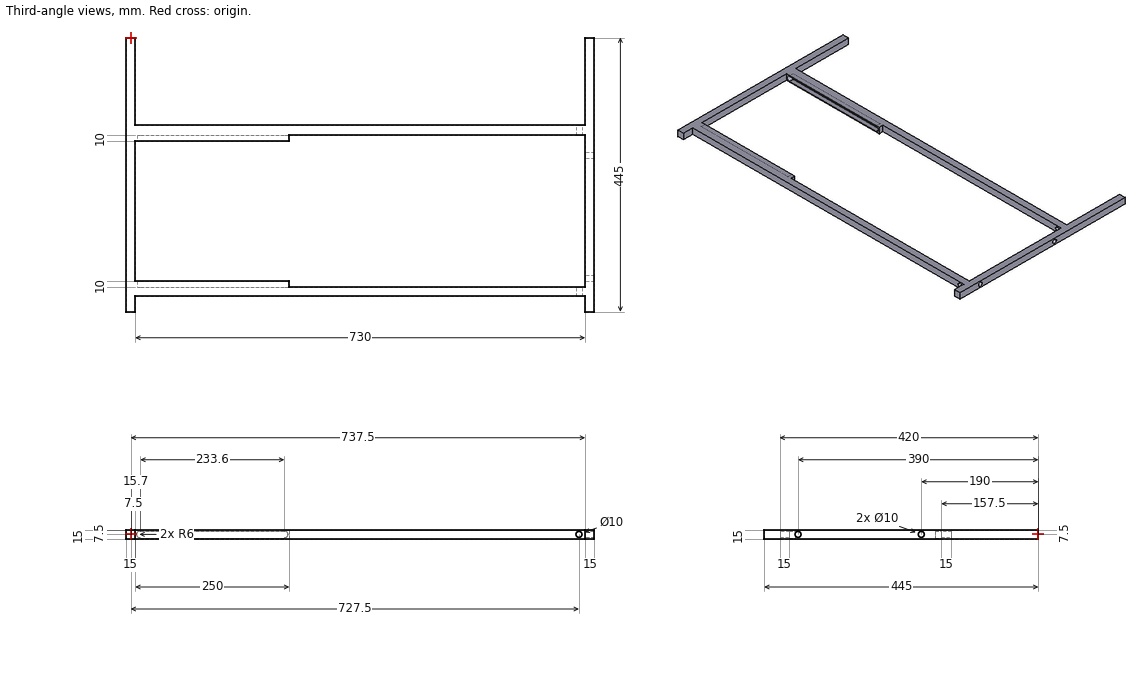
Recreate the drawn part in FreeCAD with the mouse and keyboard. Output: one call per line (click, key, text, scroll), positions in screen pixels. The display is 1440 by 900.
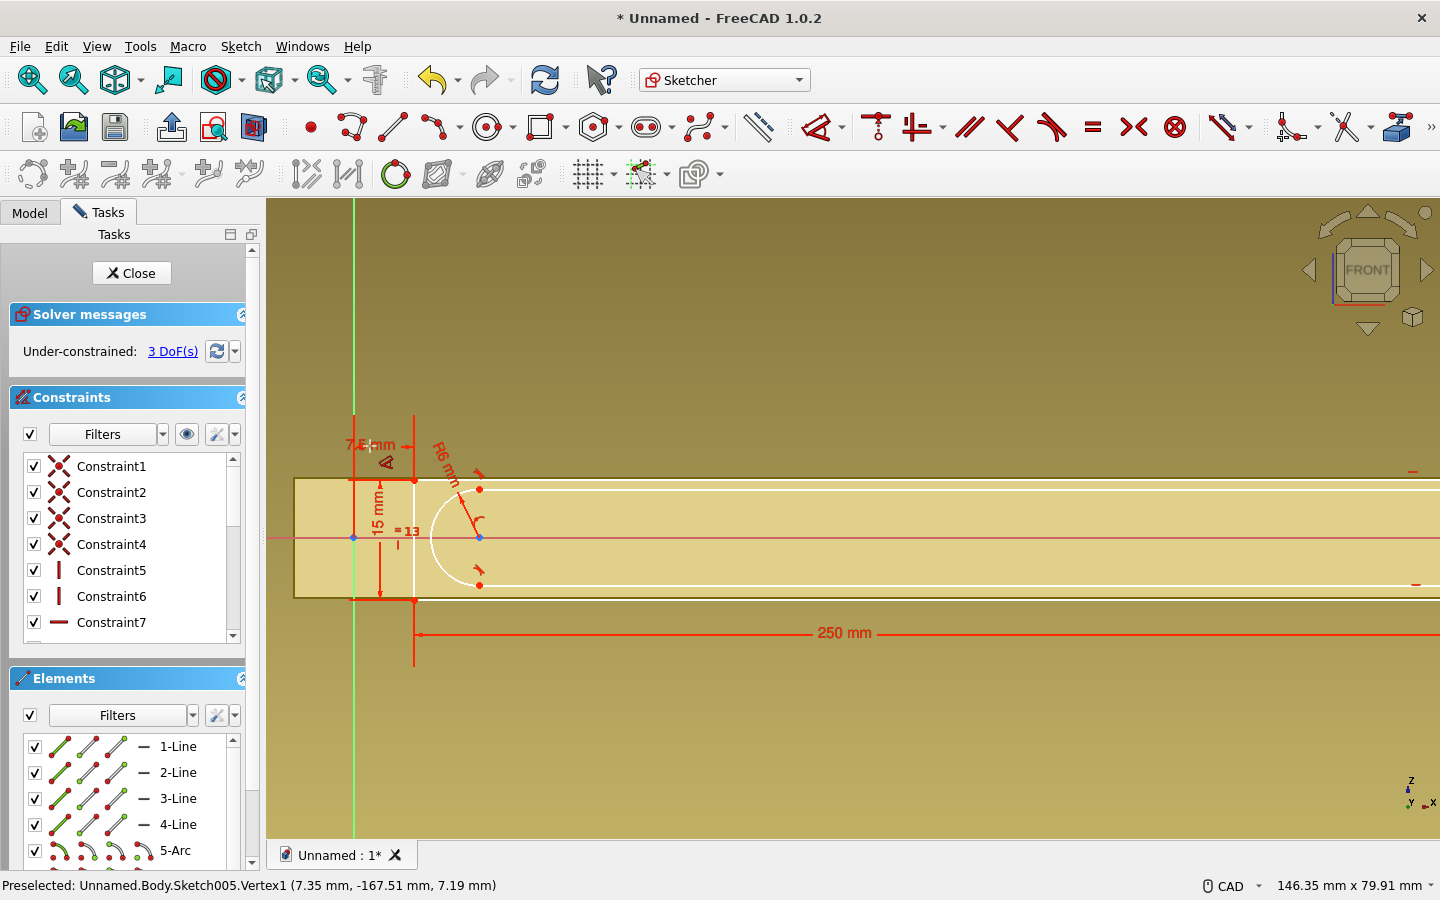
click(414, 480)
click(320, 489)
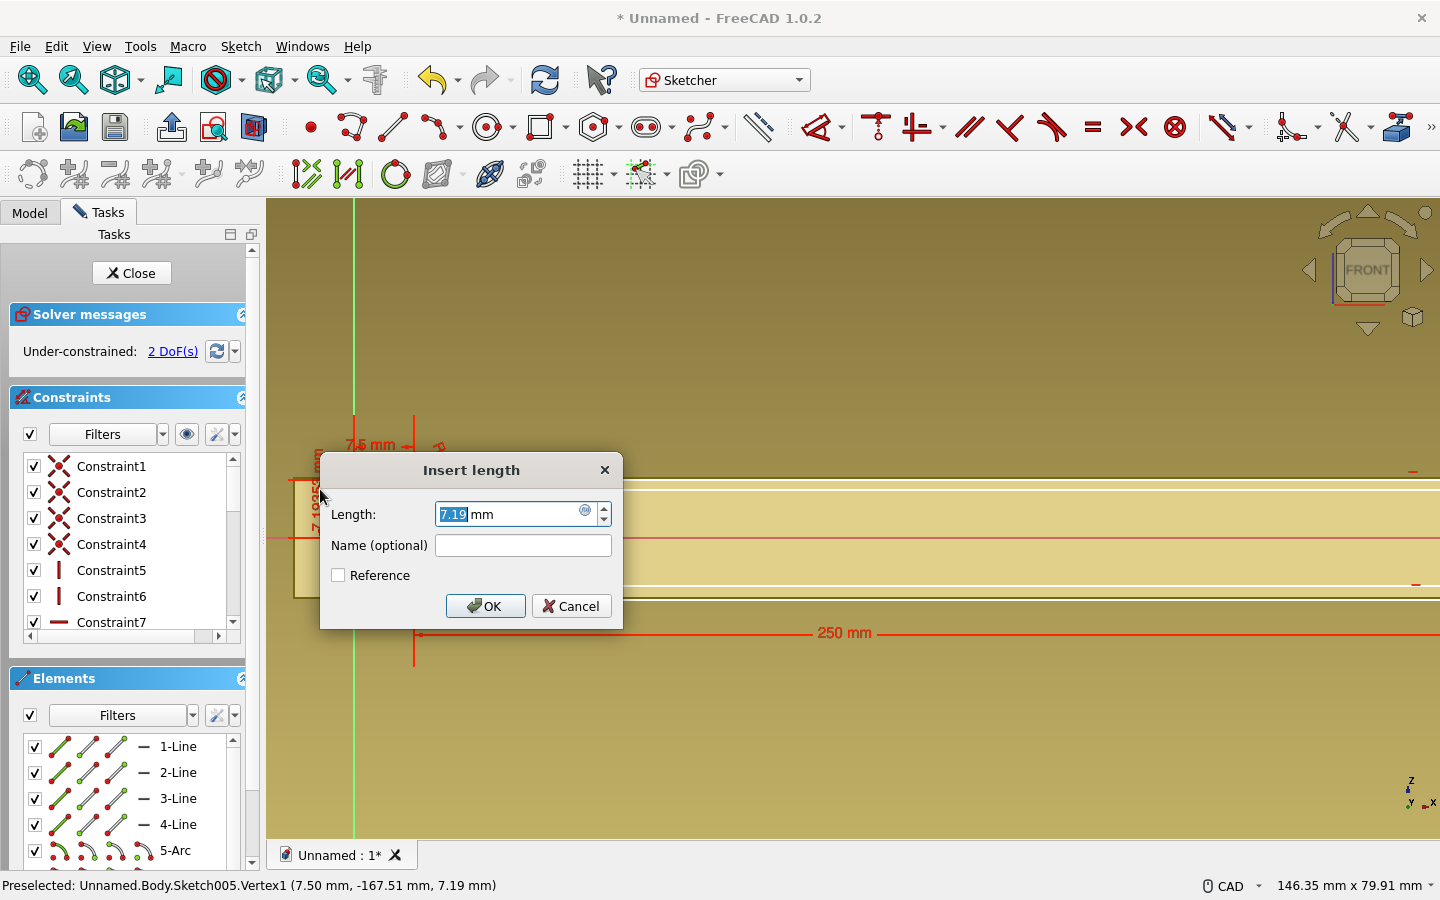
text(7.5)
key(Return)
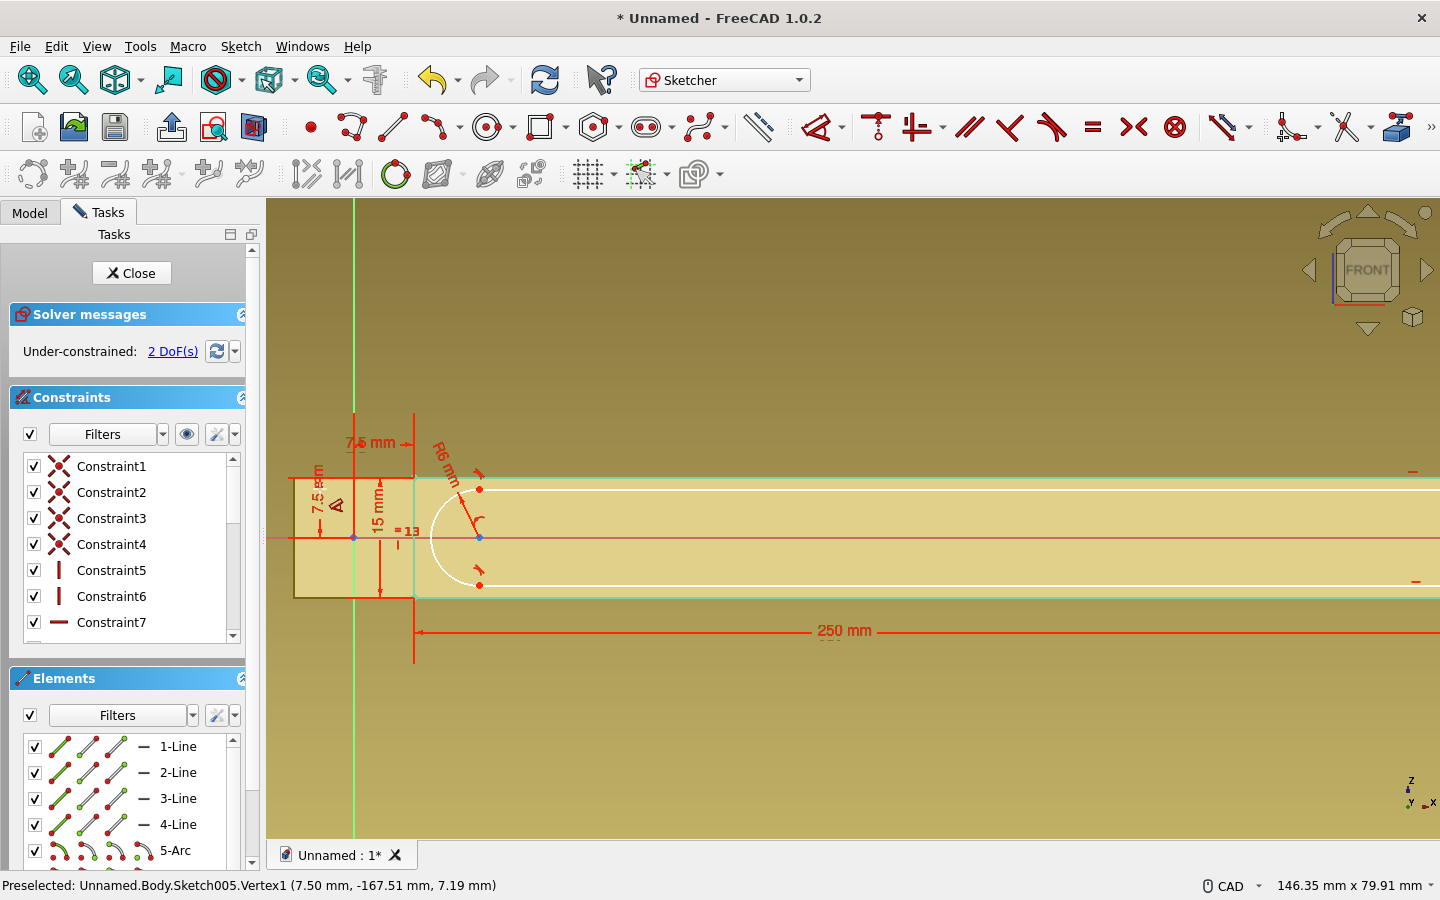
click(1041, 490)
click(877, 456)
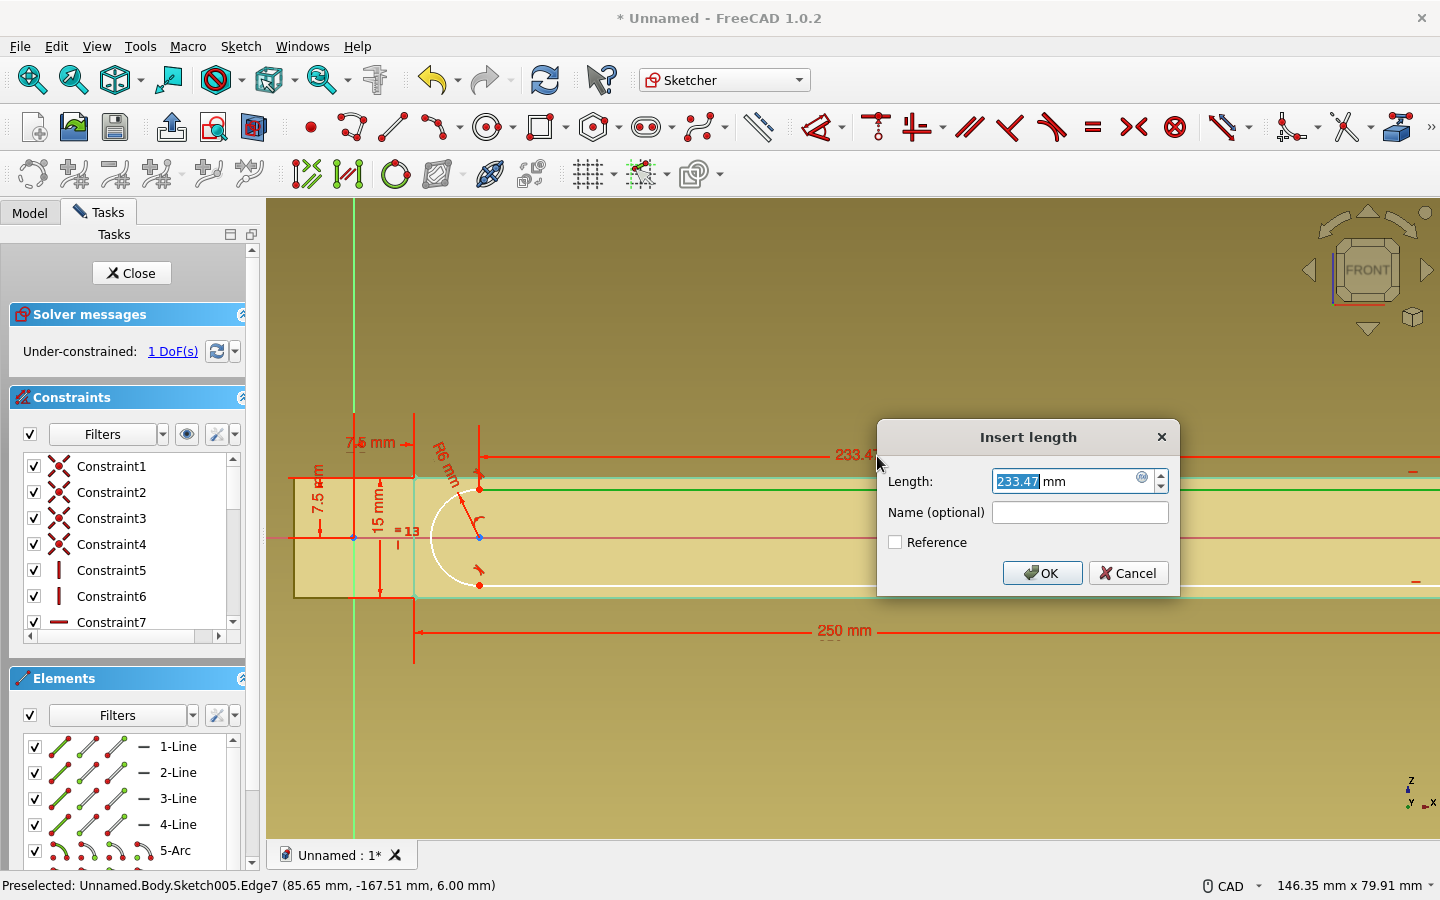
text(233.6)
key(Return)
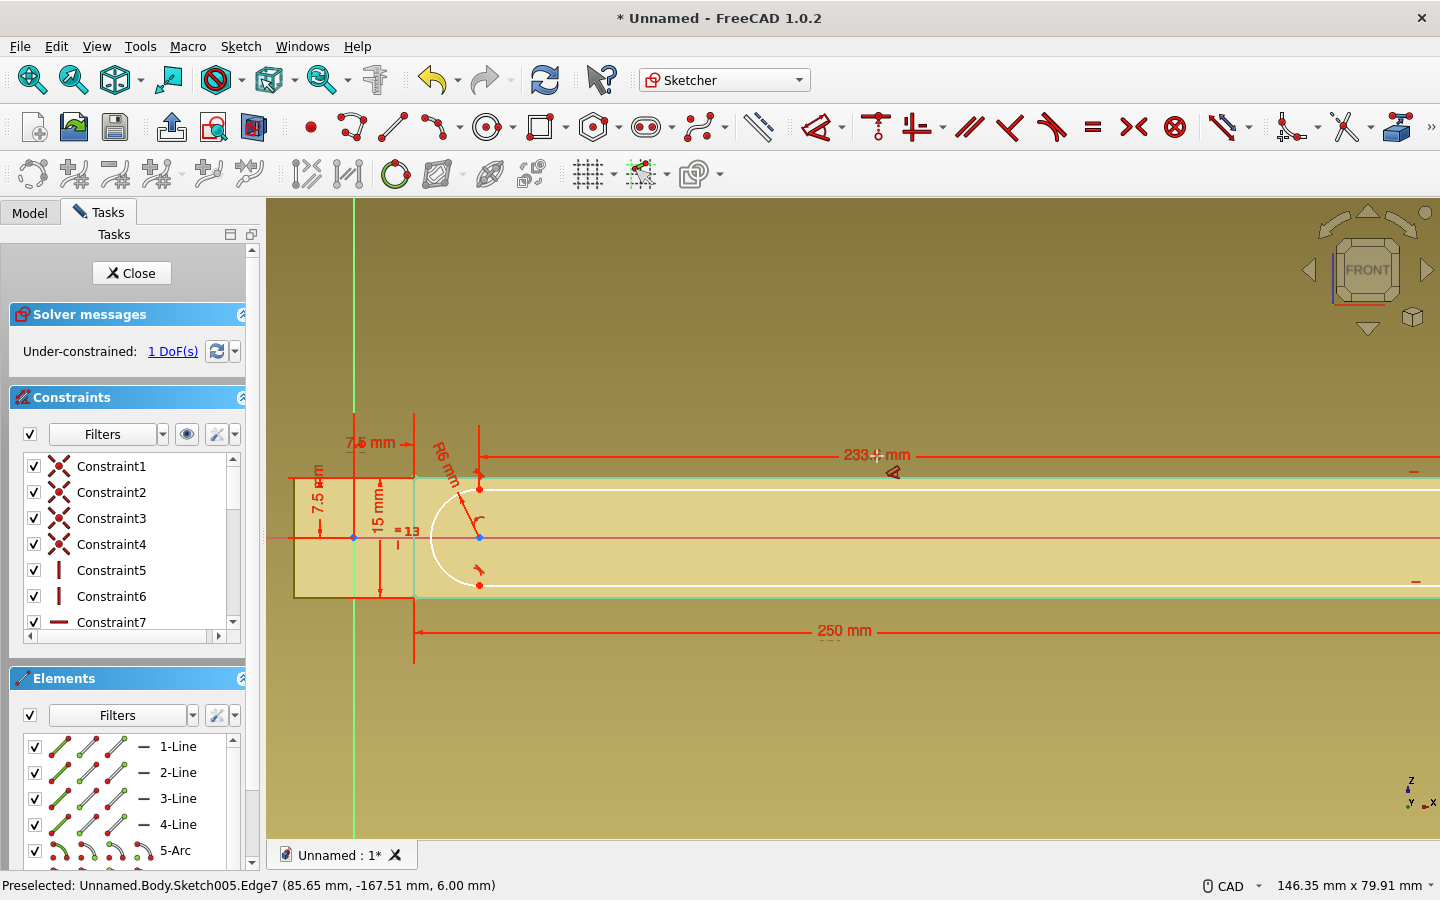
click(479, 490)
click(388, 572)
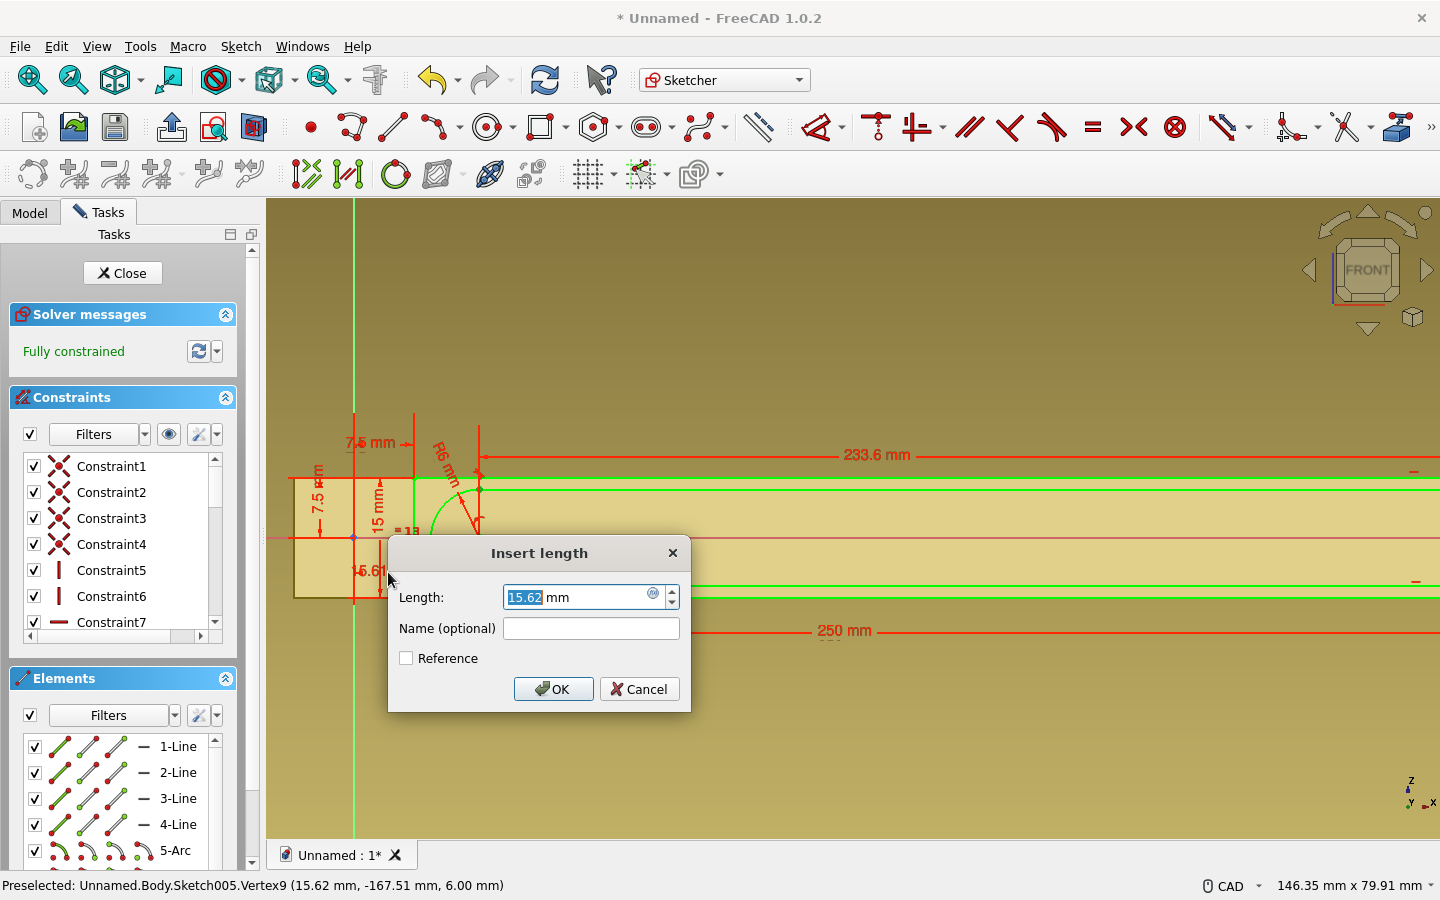
text(15.7)
key(Return)
key(Escape)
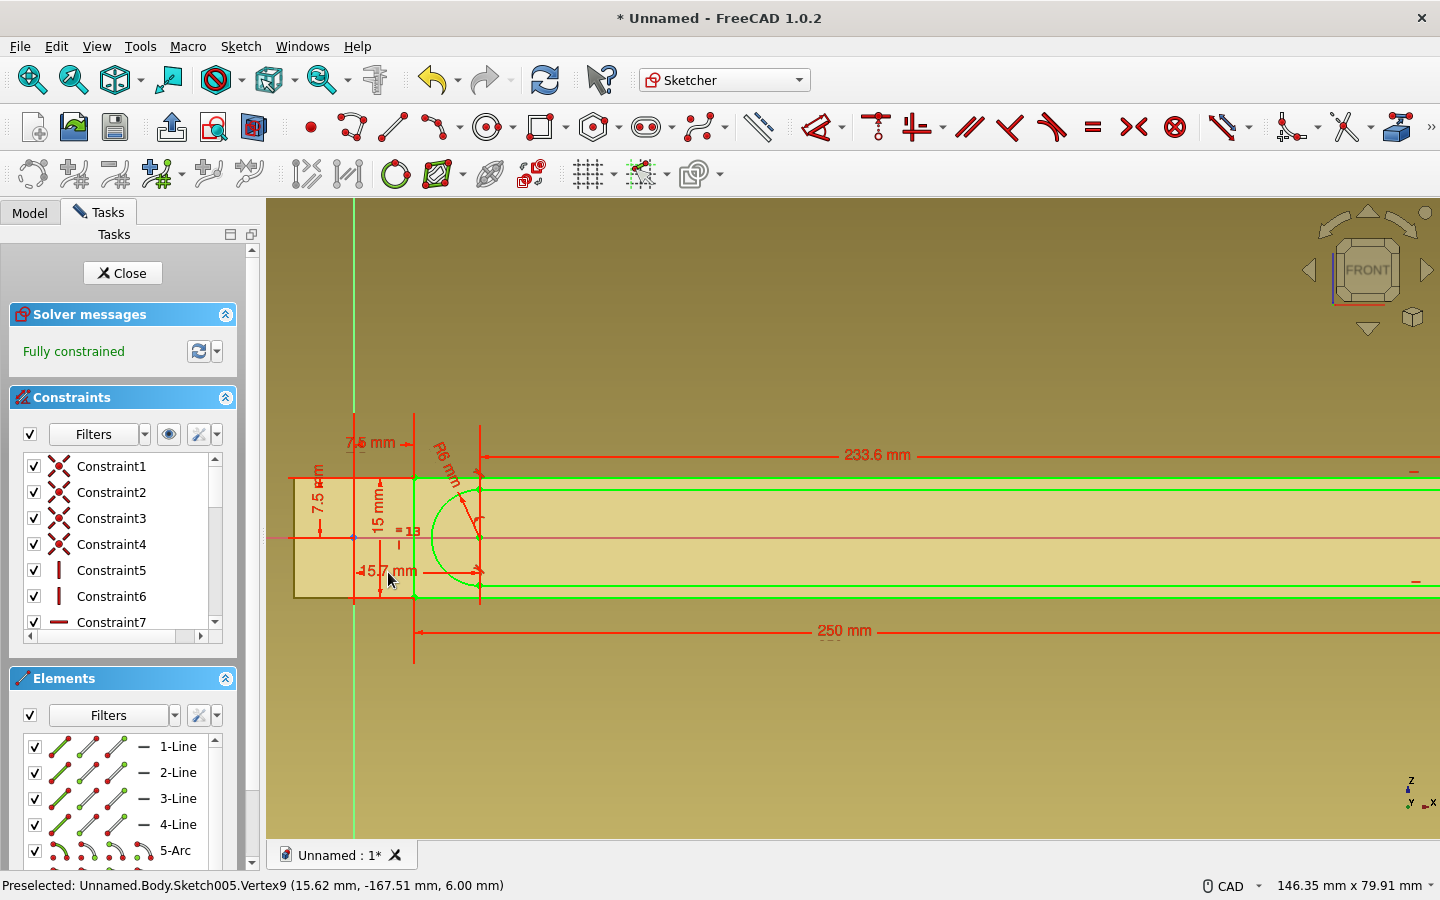
click(123, 273)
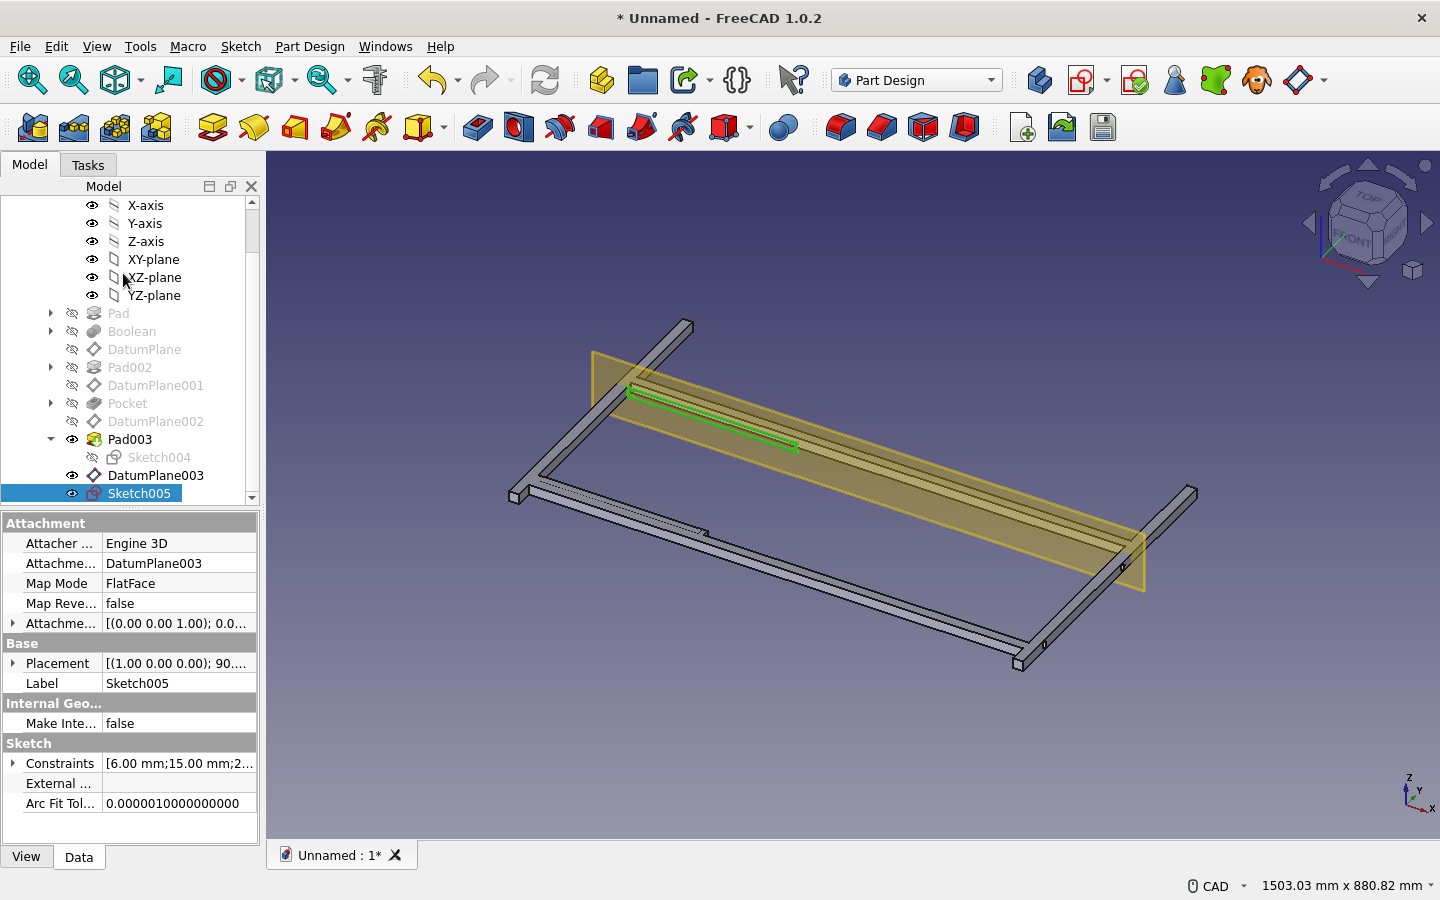
click(213, 128)